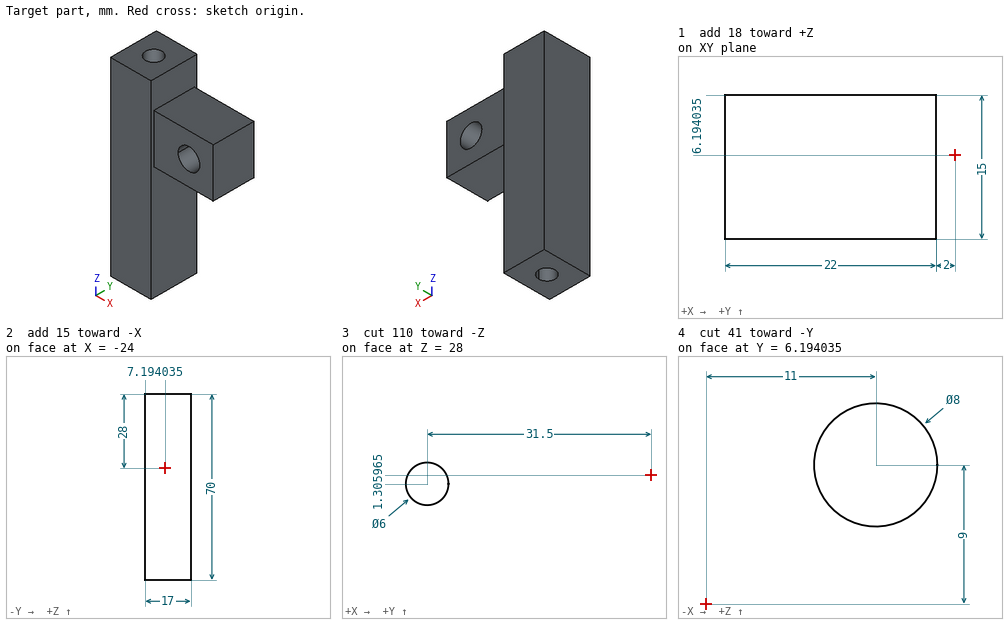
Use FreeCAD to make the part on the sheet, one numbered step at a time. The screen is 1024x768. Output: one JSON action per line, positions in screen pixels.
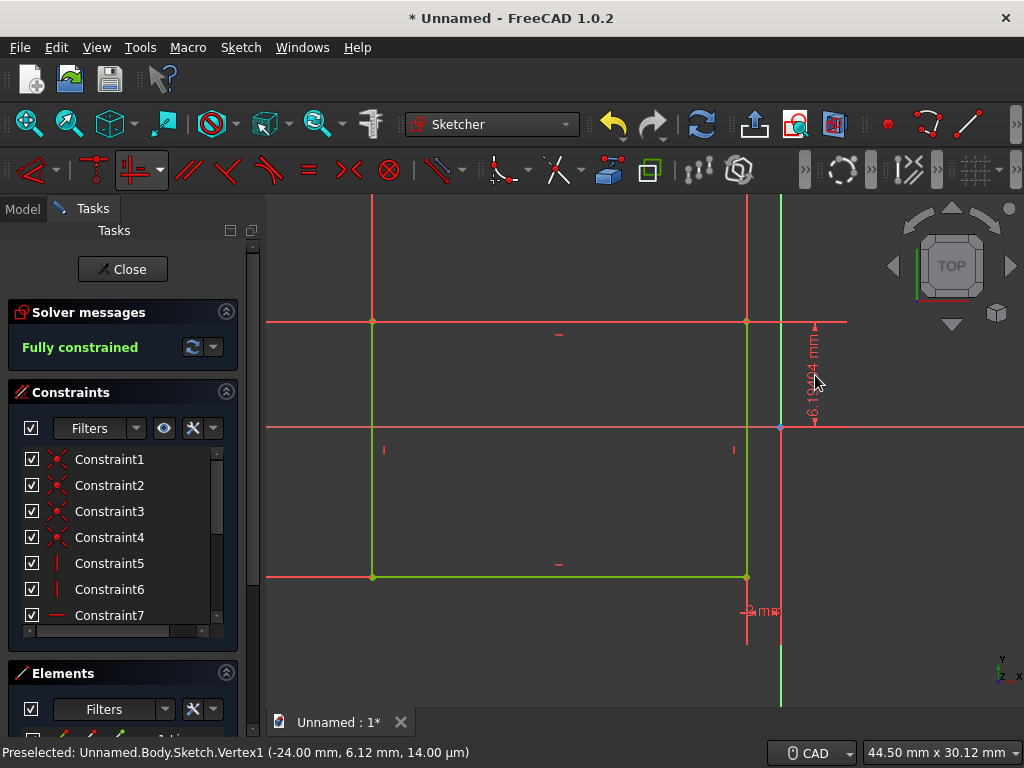
{"action": "left_click", "coordinate": [123, 269]}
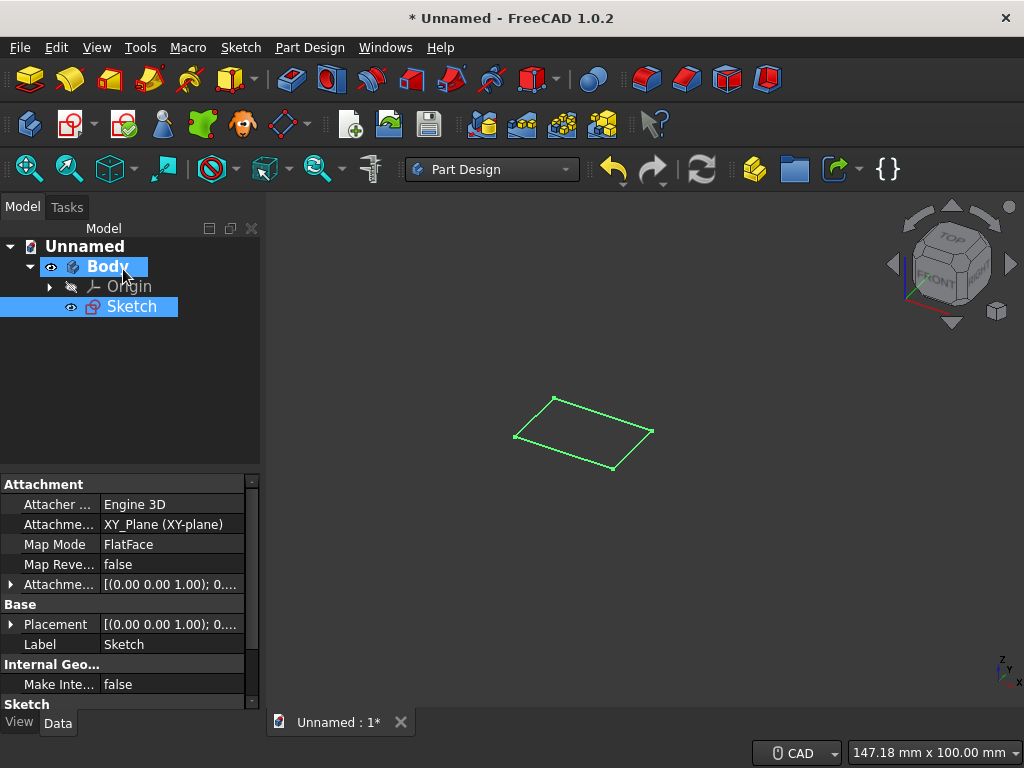
{"action": "left_click", "coordinate": [30, 80]}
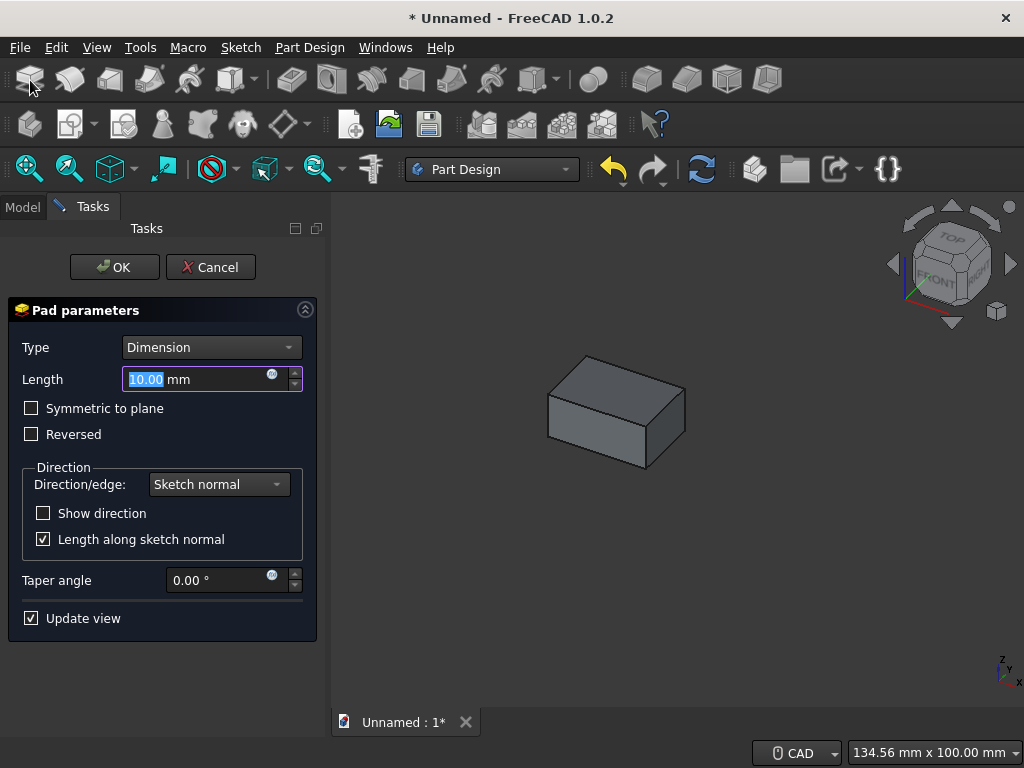
{"action": "type", "text": "18"}
{"action": "key", "text": "Tab"}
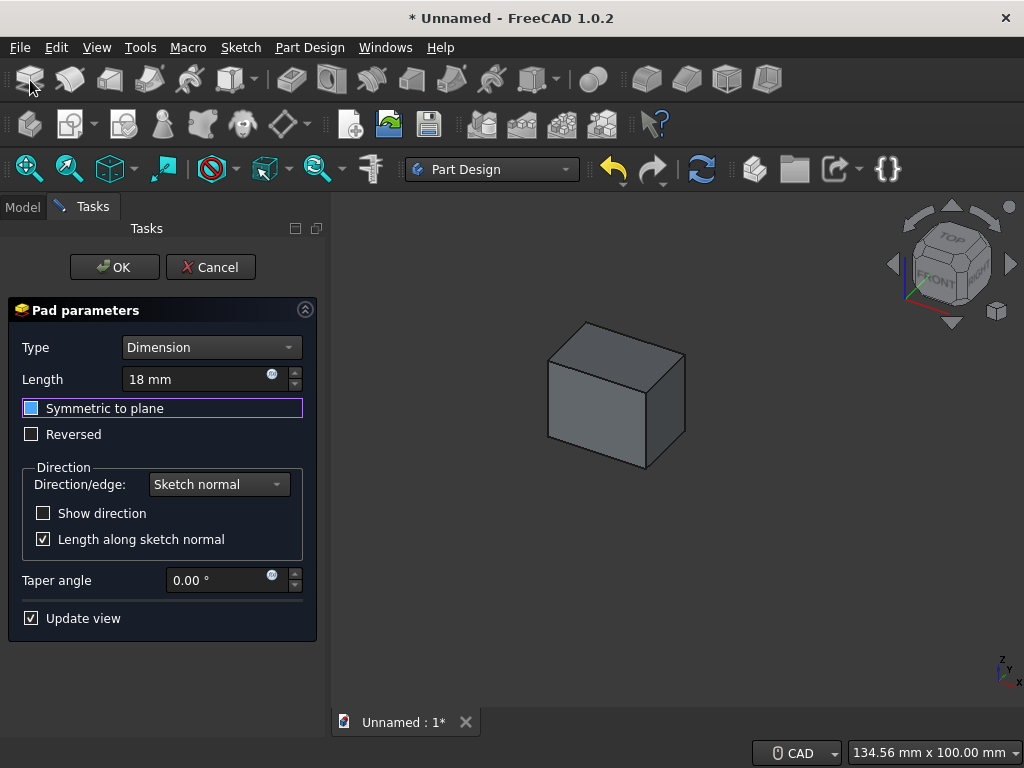
{"action": "left_click", "coordinate": [115, 267]}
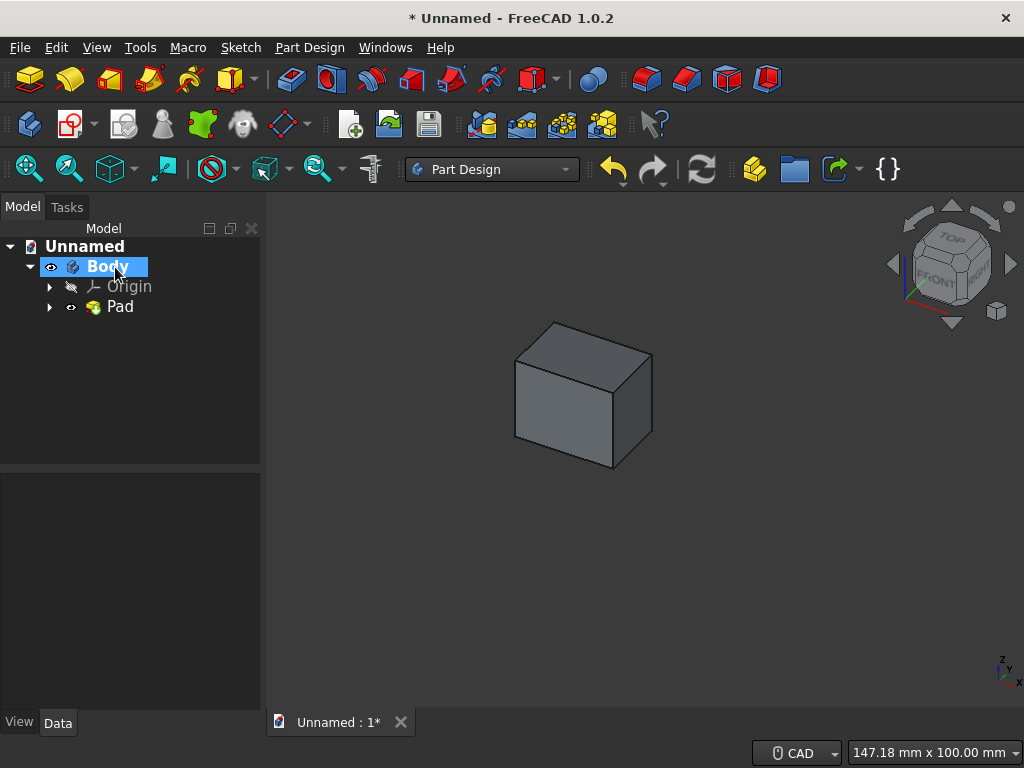
{"action": "left_click", "coordinate": [30, 170]}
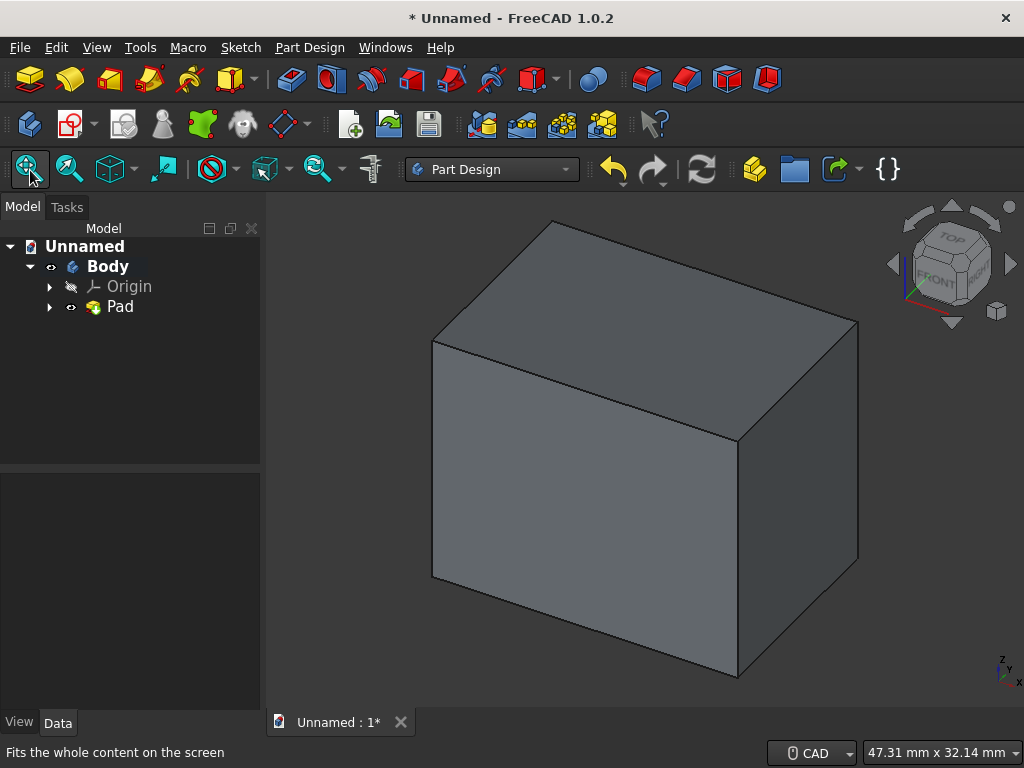
{"action": "key", "text": "6"}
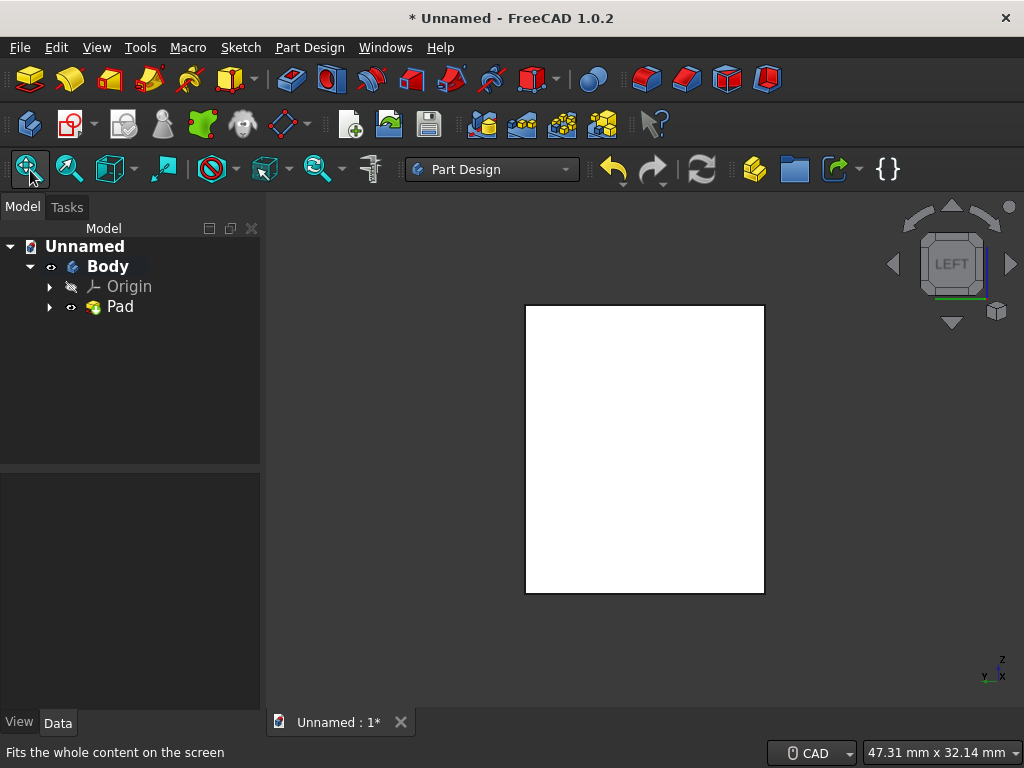
{"action": "left_click", "coordinate": [645, 448]}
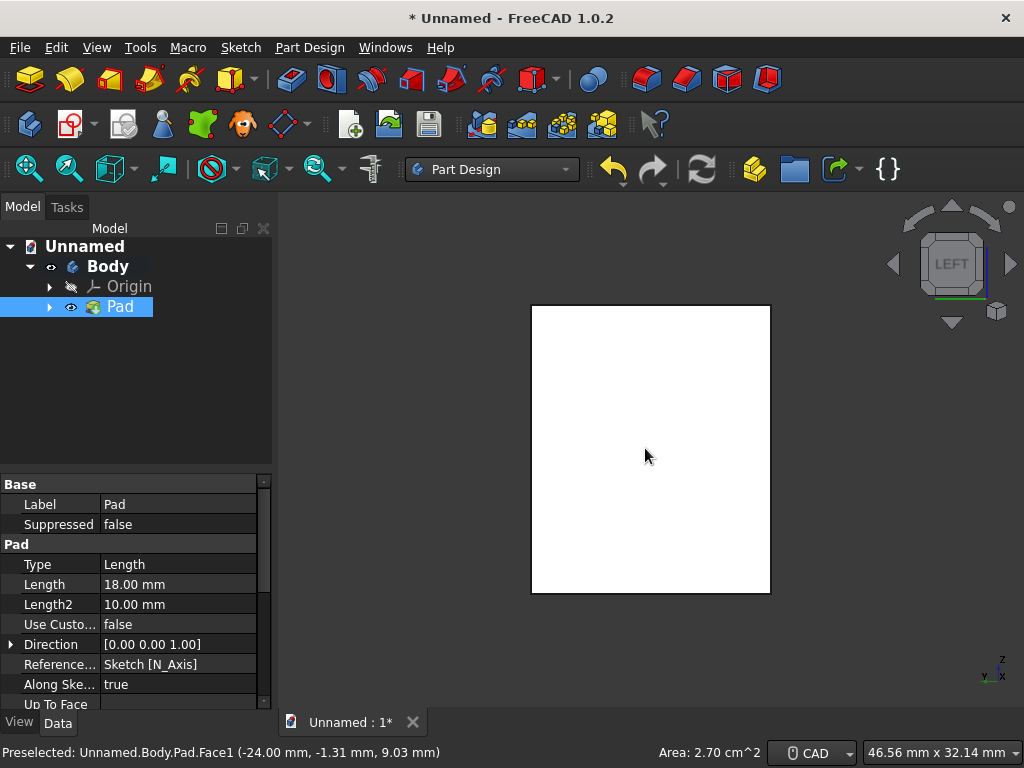
{"action": "left_click", "coordinate": [70, 124]}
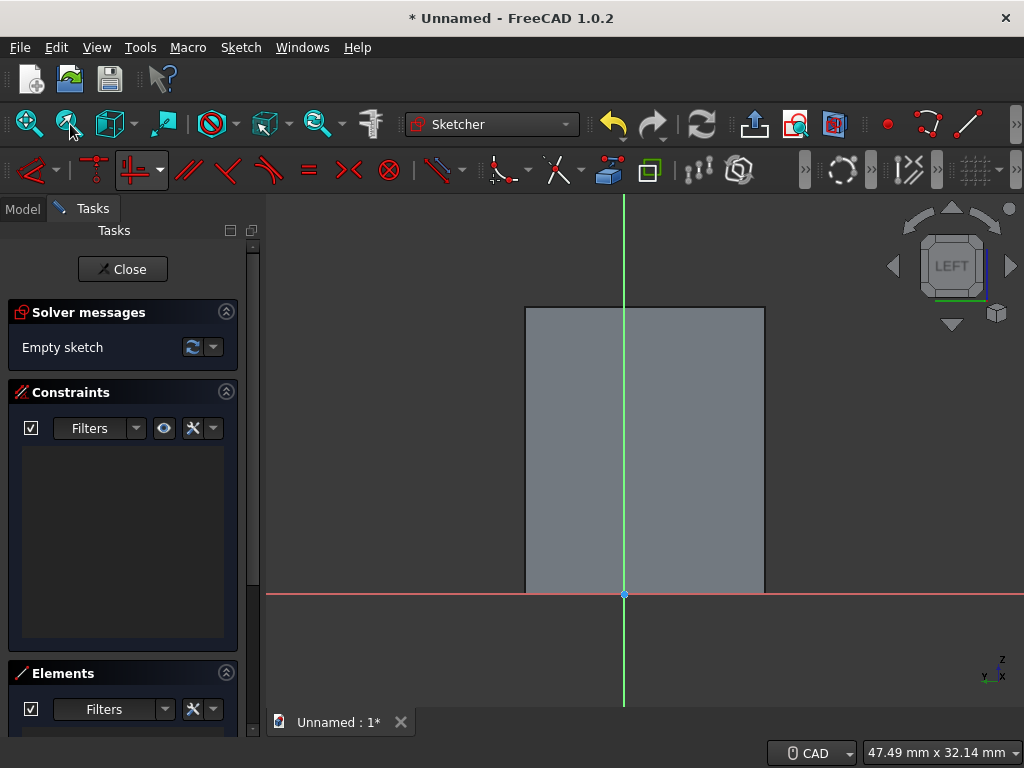
{"action": "scroll", "coordinate": [547, 340], "scroll_direction": "down", "scroll_amount": 6}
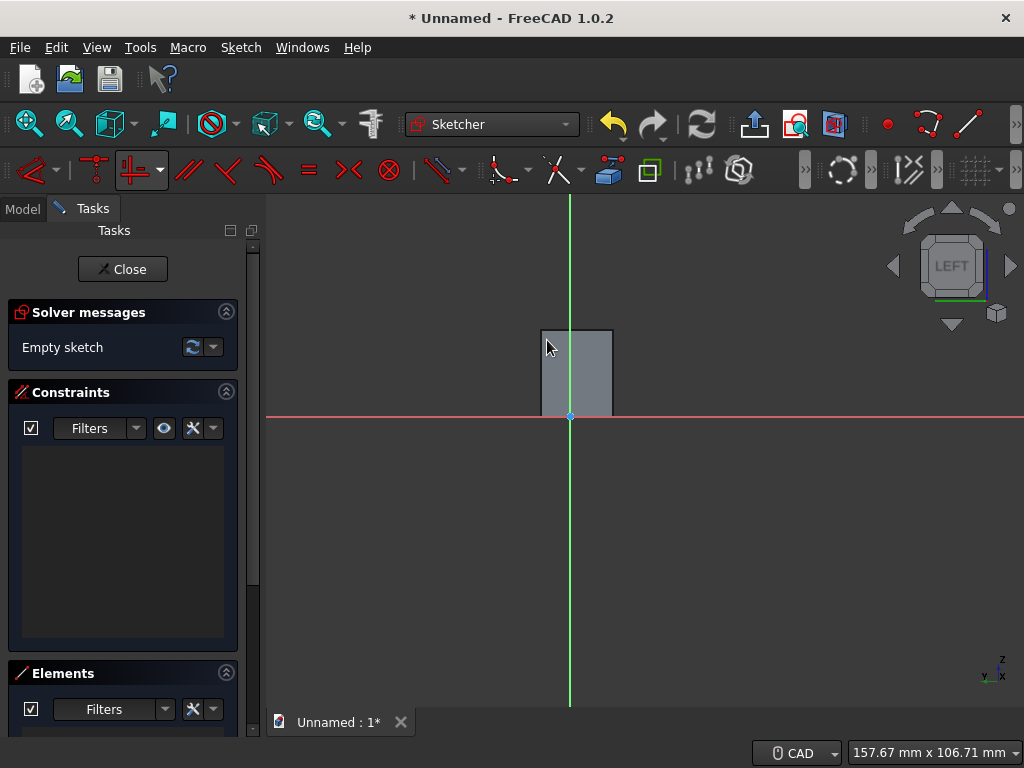
{"action": "key", "text": "g r"}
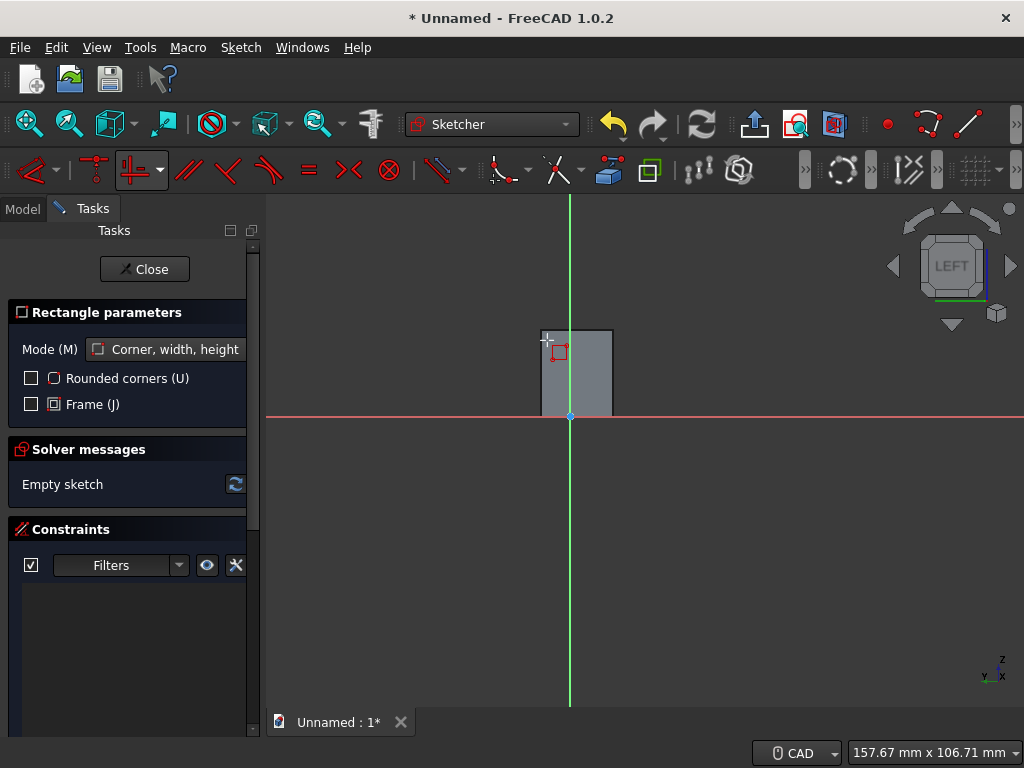
{"action": "left_click", "coordinate": [536, 282]}
{"action": "mouse_move", "coordinate": [618, 619]}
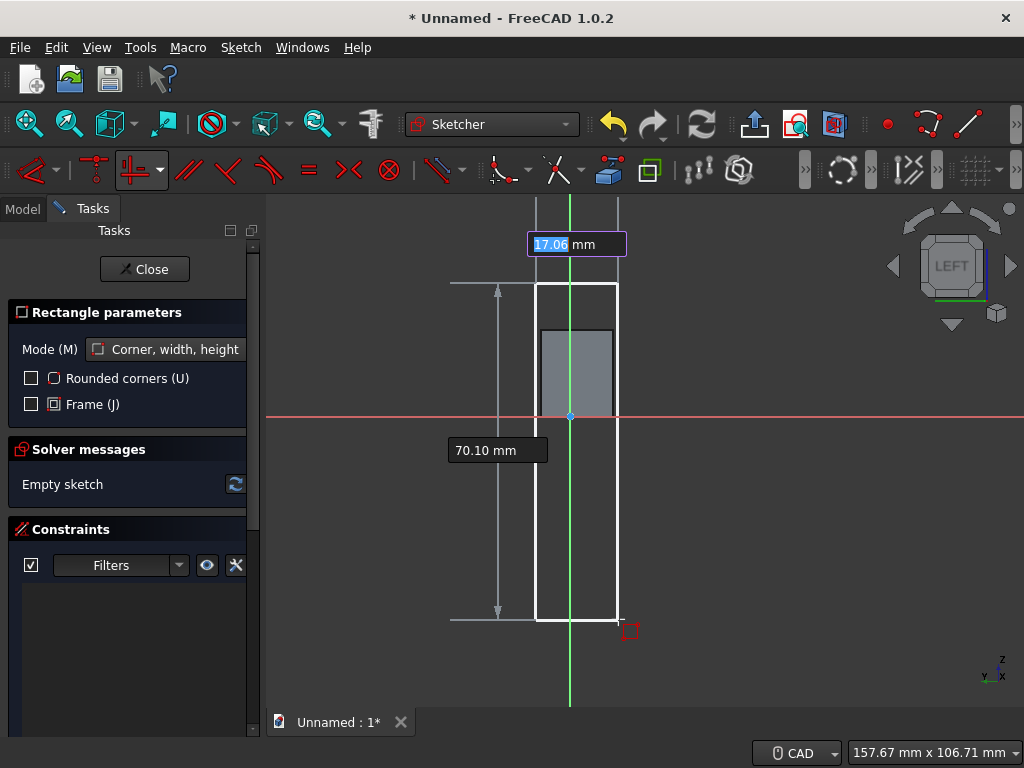
{"action": "type", "text": "17"}
{"action": "key", "text": "Tab"}
{"action": "type", "text": "70"}
{"action": "key", "text": "Return"}
{"action": "key", "text": "Escape"}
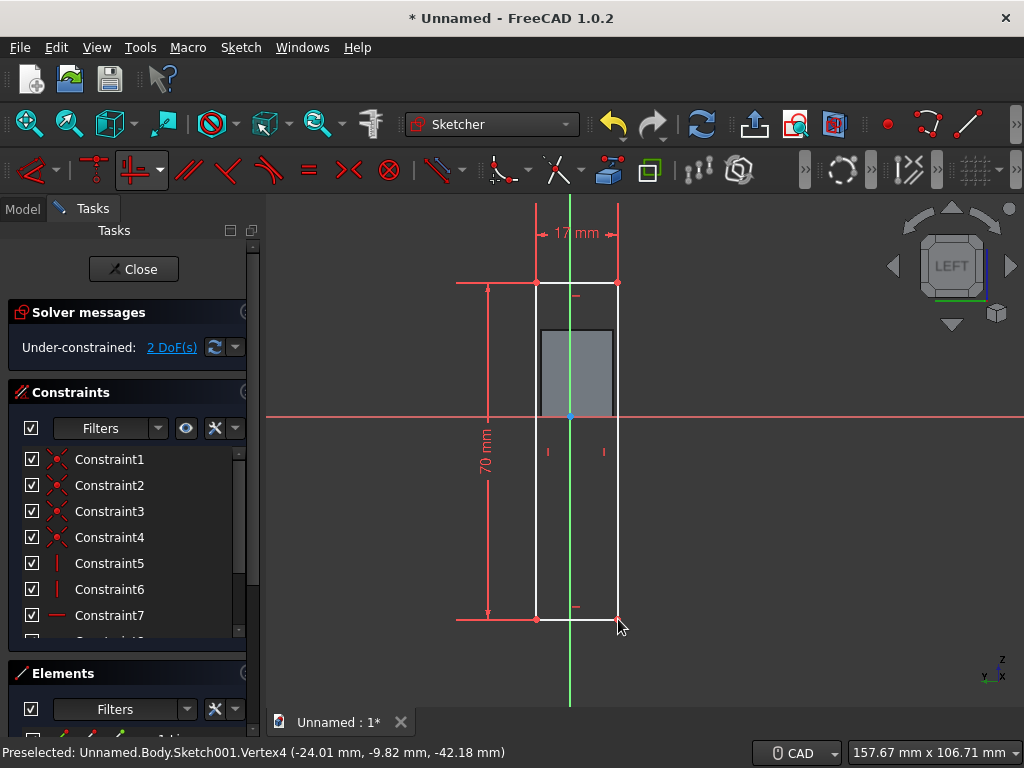
{"action": "left_click", "coordinate": [32, 170]}